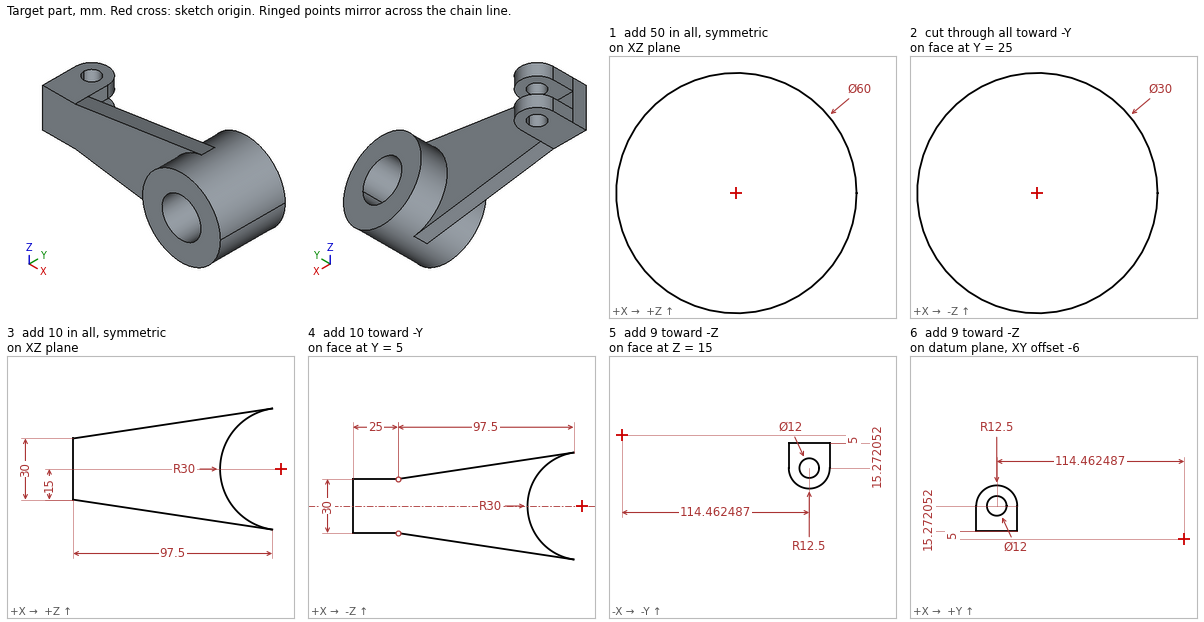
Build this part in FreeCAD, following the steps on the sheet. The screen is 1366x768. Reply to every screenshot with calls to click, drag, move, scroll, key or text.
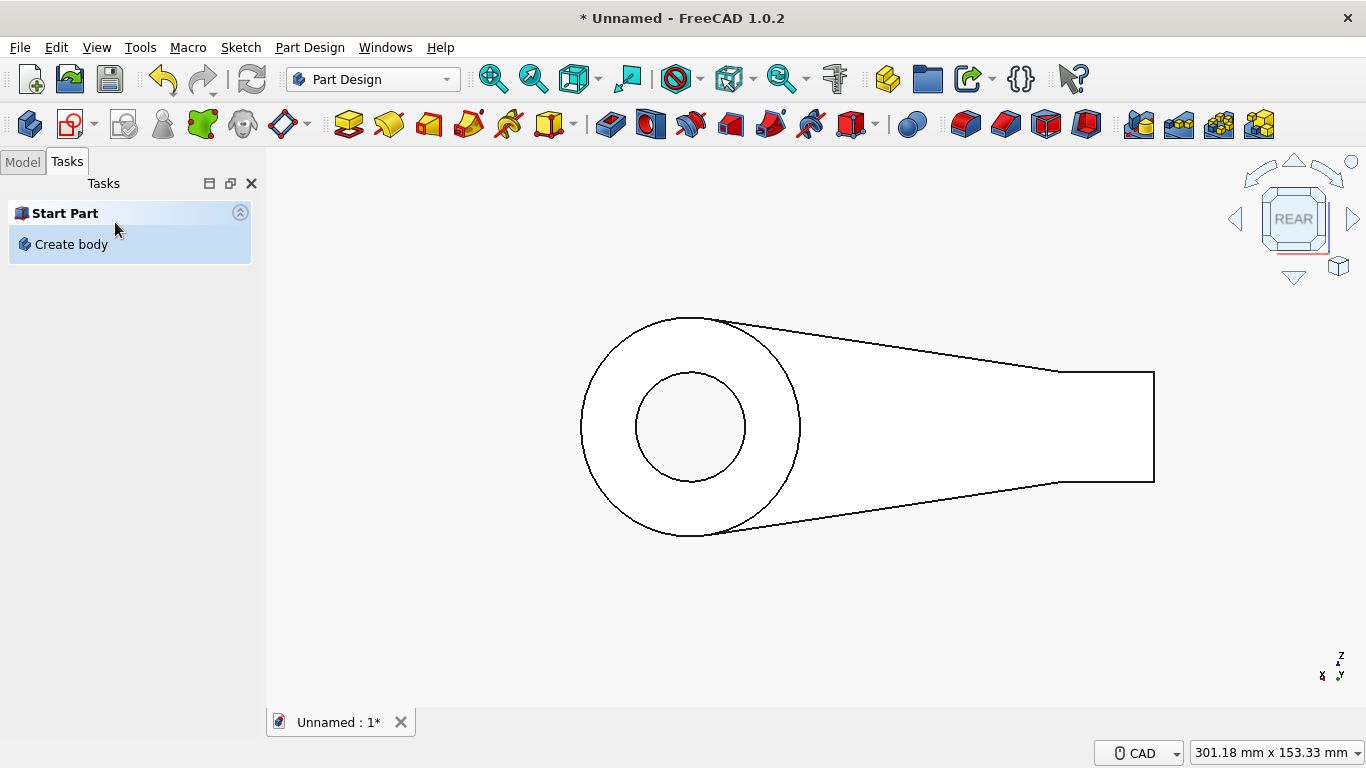
key(0)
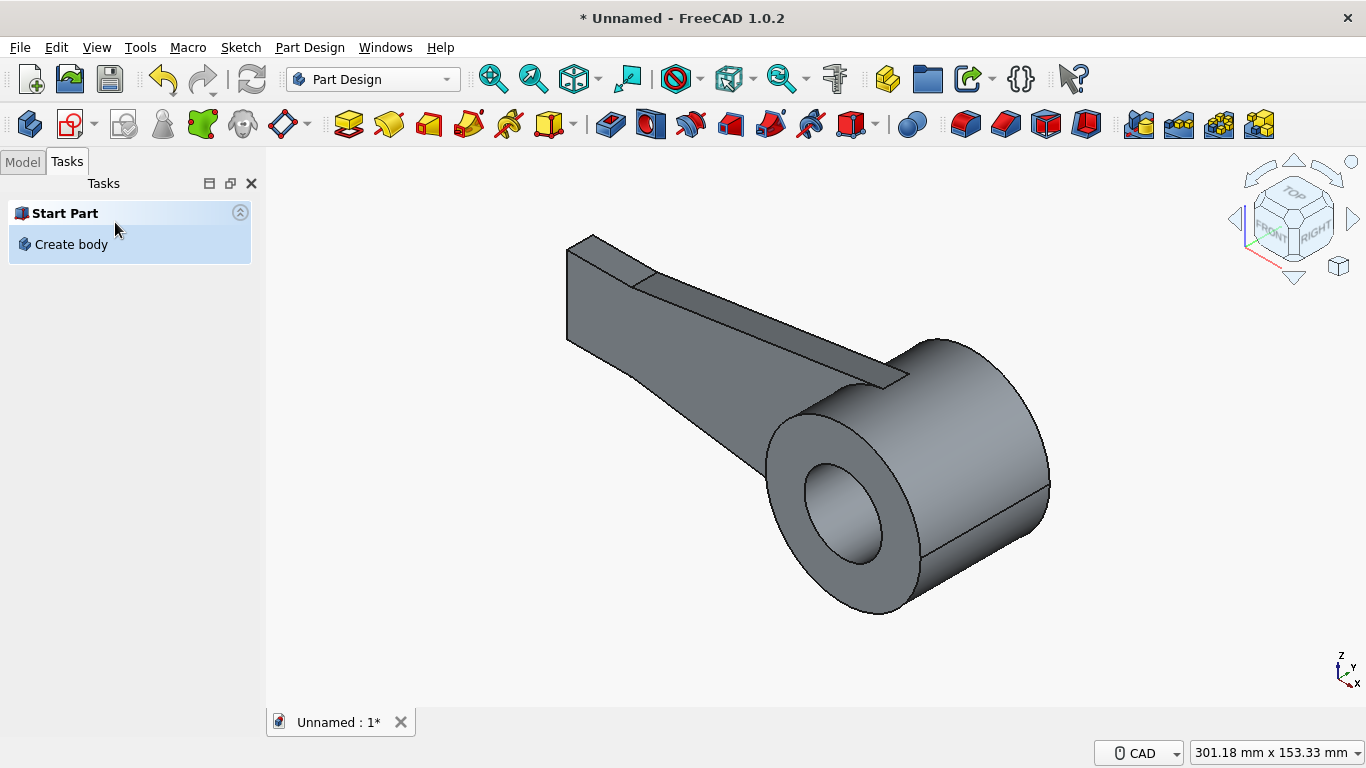
click(631, 271)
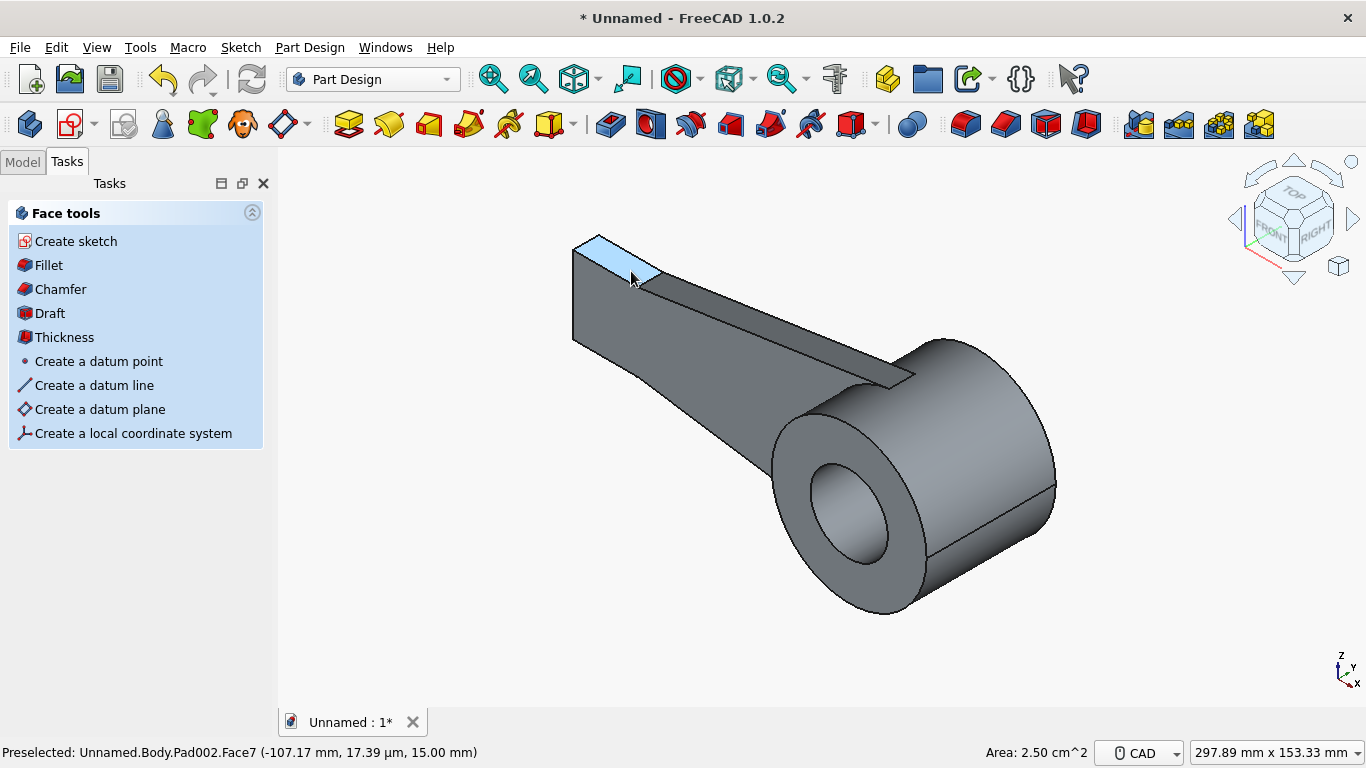
click(70, 124)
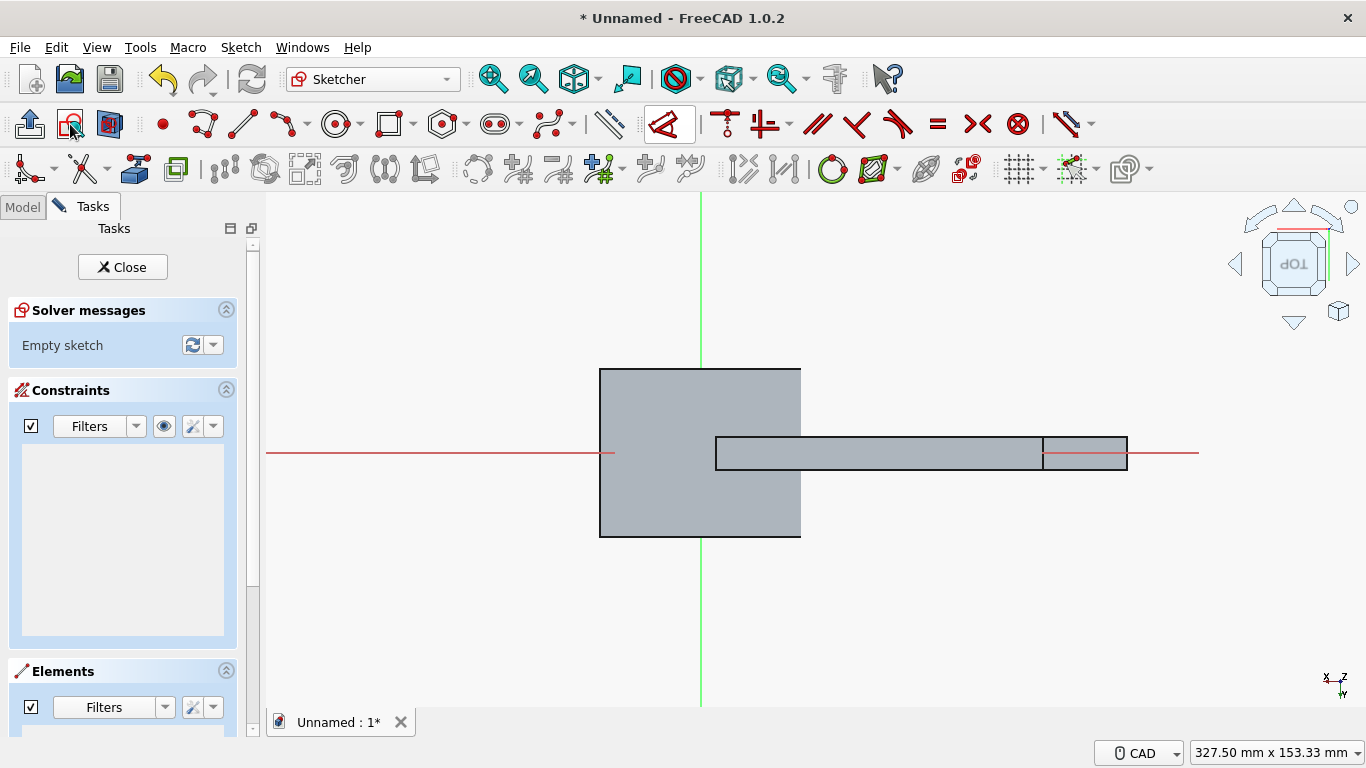
click(110, 124)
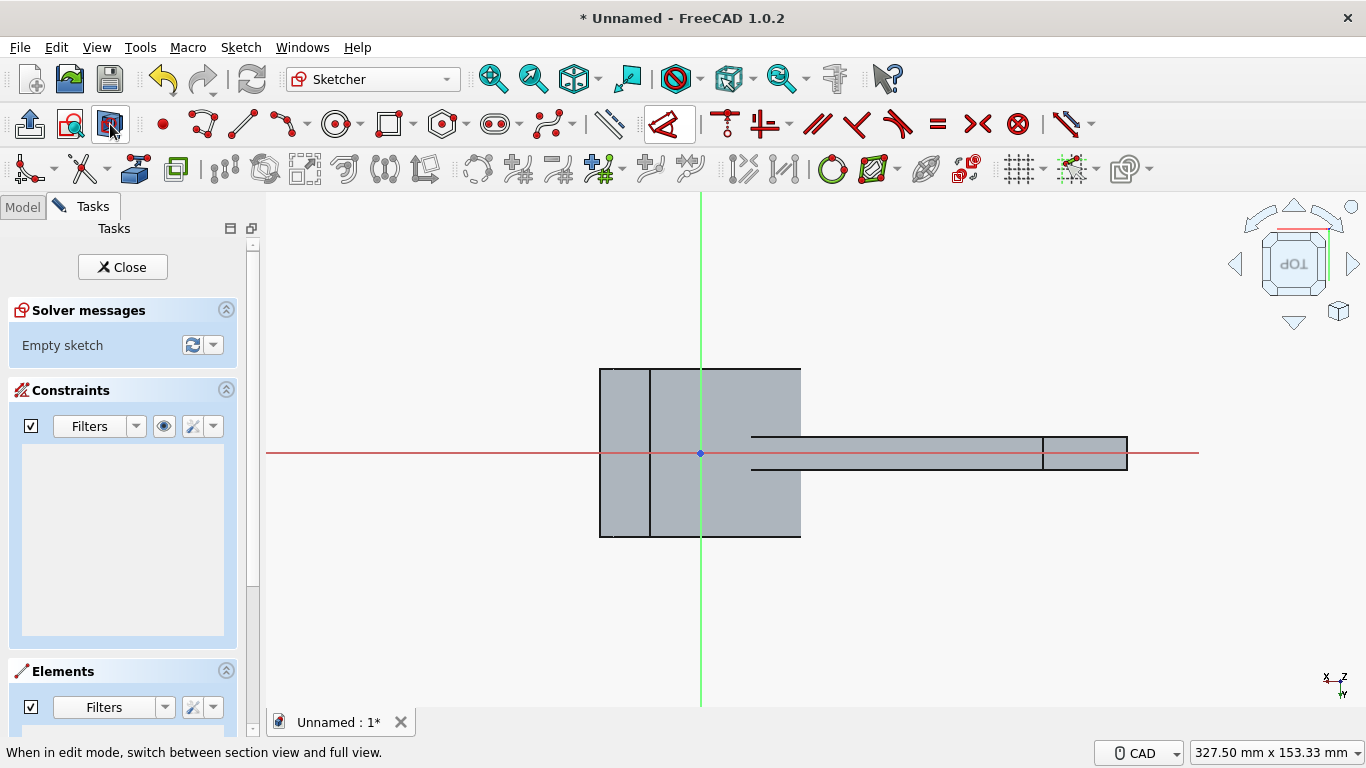
scroll(1201, 546, up, 6)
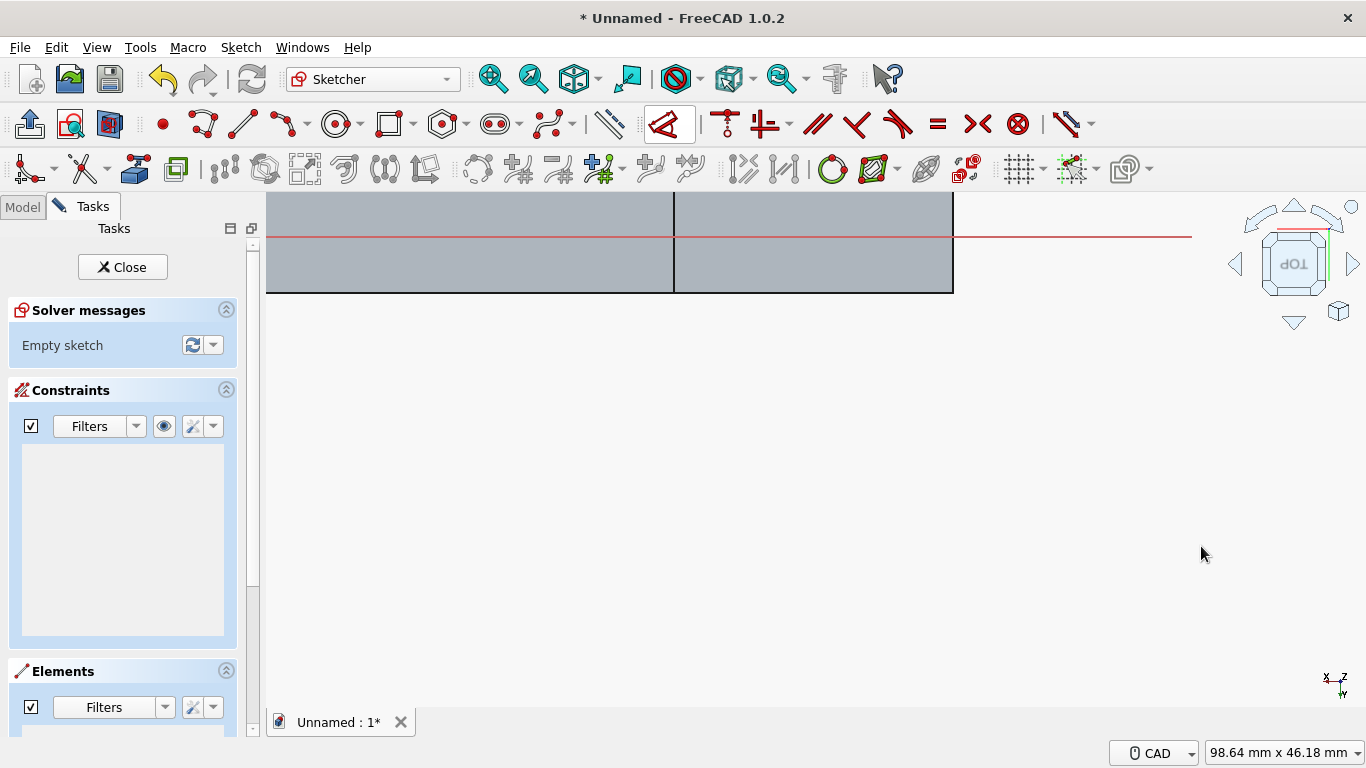
click(204, 124)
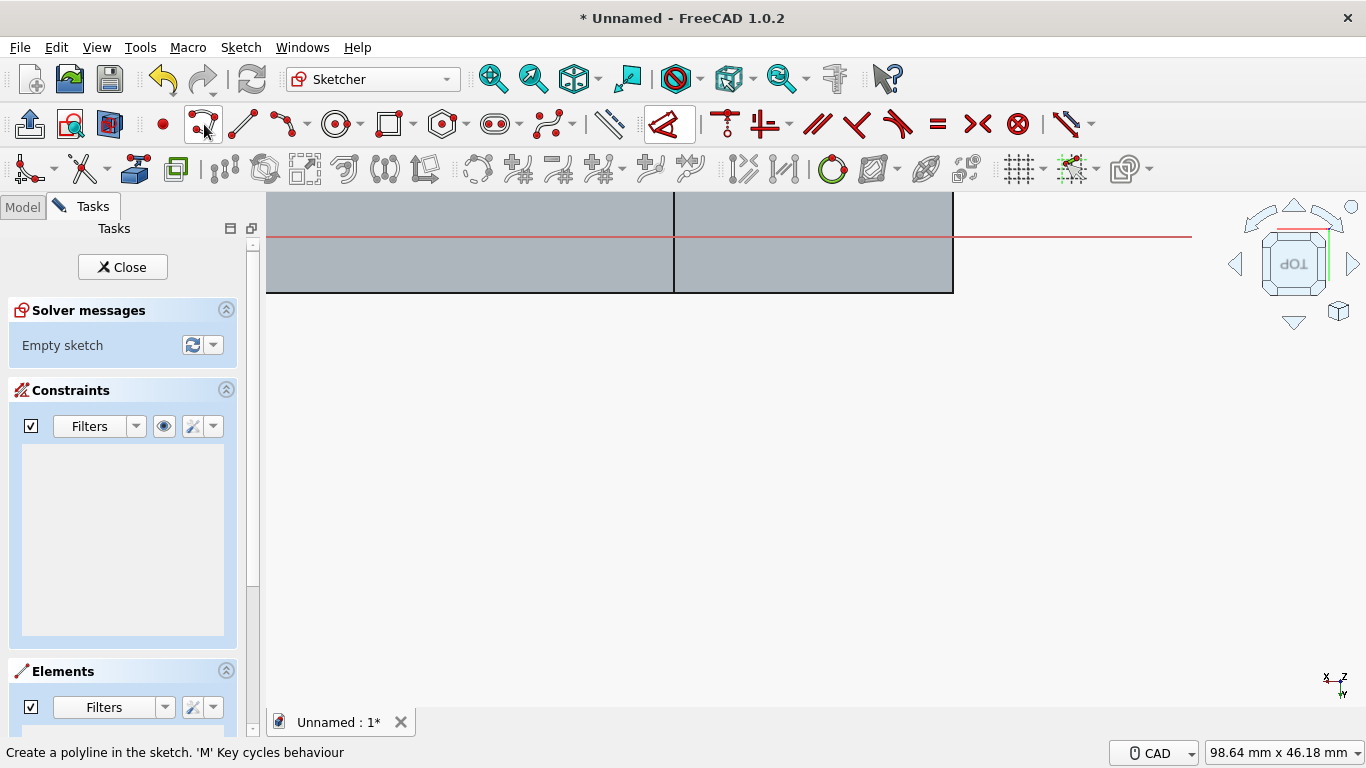
click(953, 463)
click(953, 293)
click(674, 293)
click(674, 463)
right_click(674, 463)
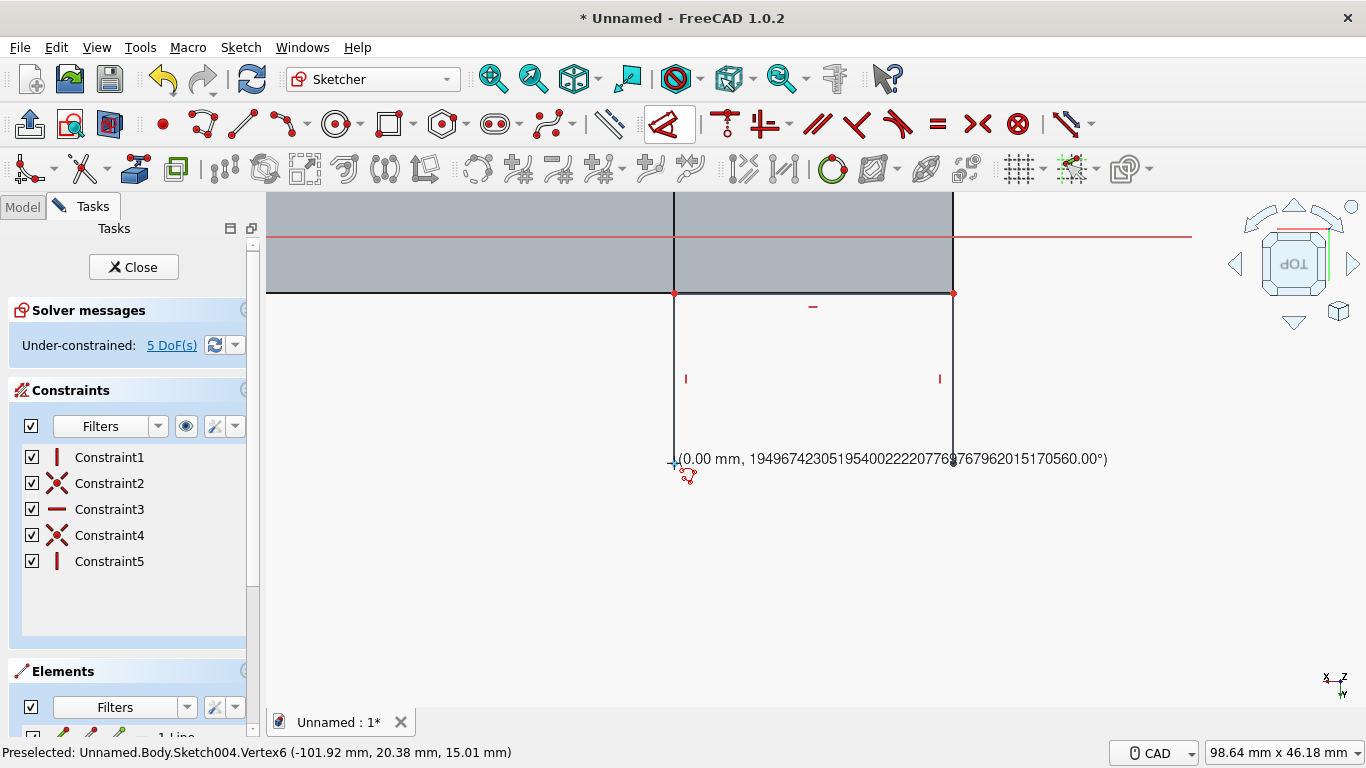
key(g)
key(3)
key(a)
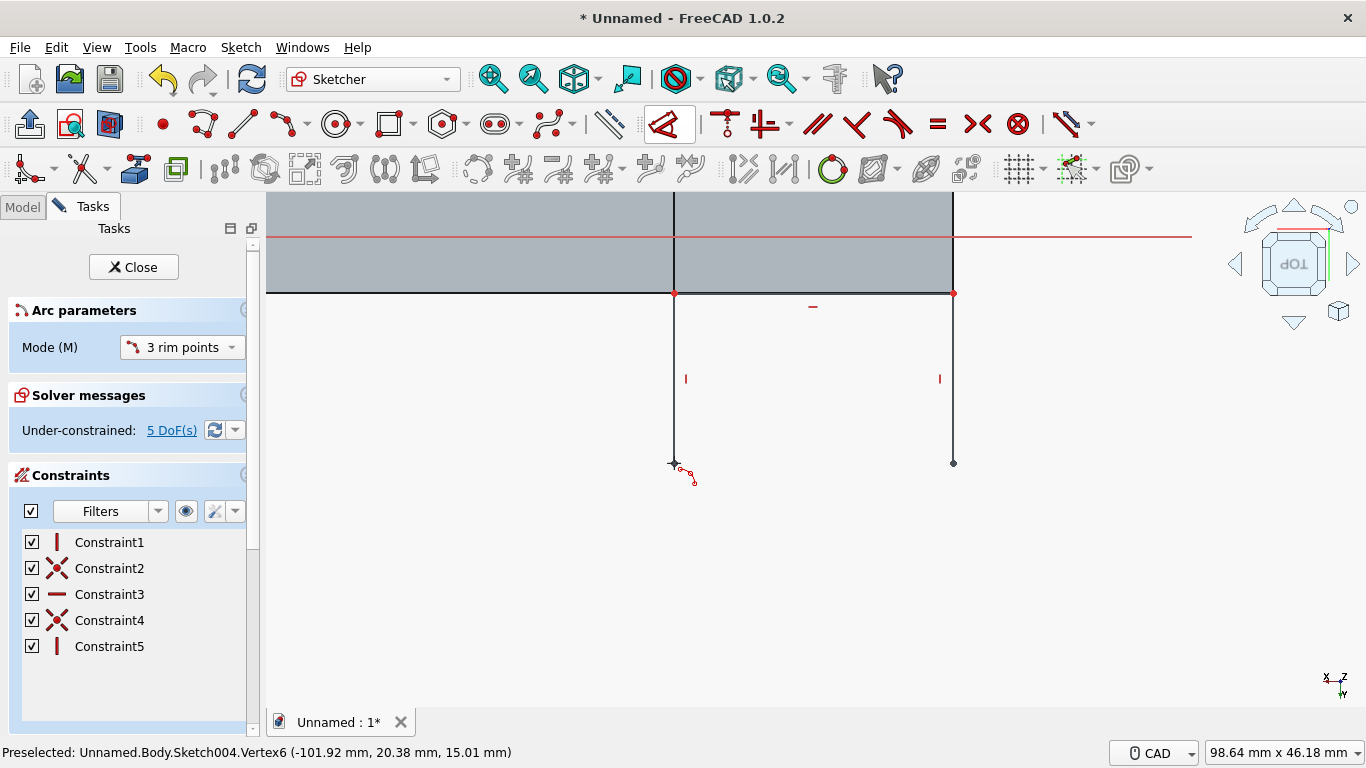
click(674, 464)
click(953, 464)
click(814, 602)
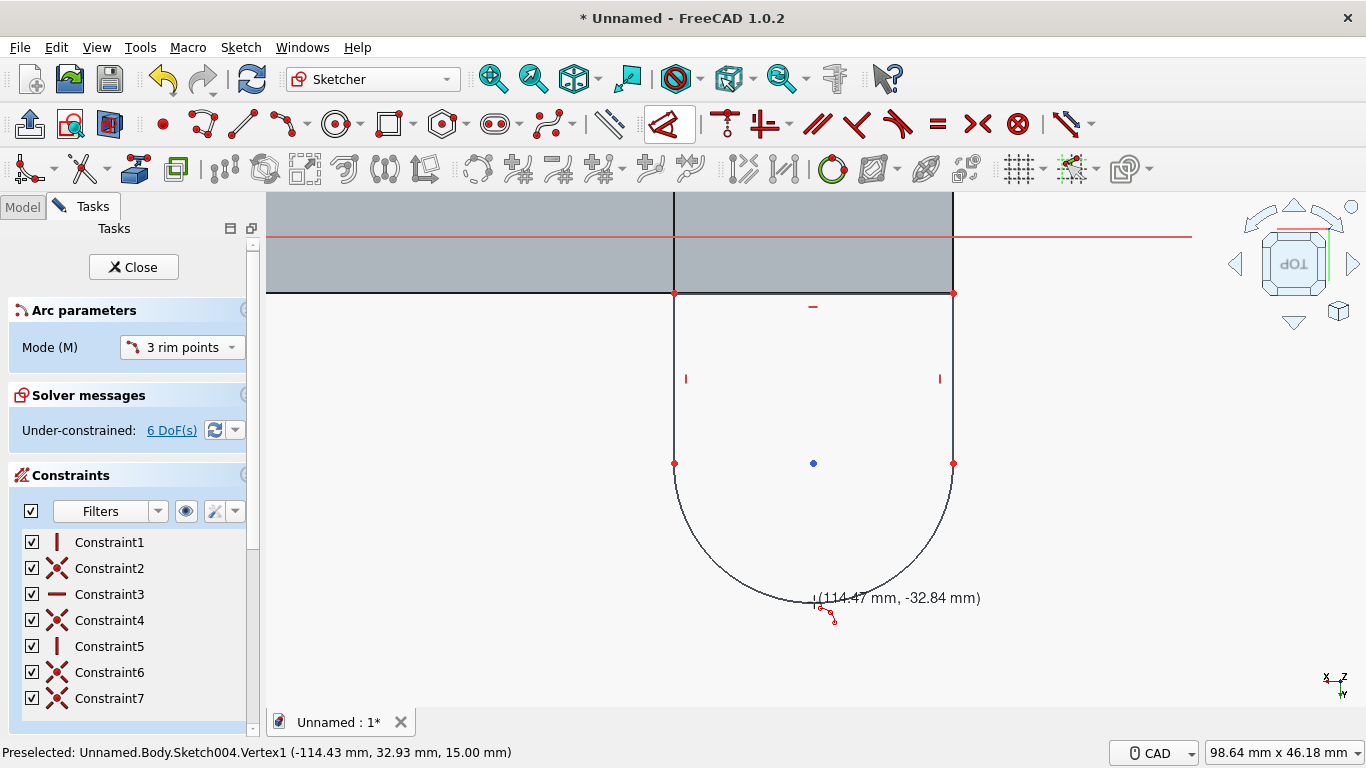
click(336, 124)